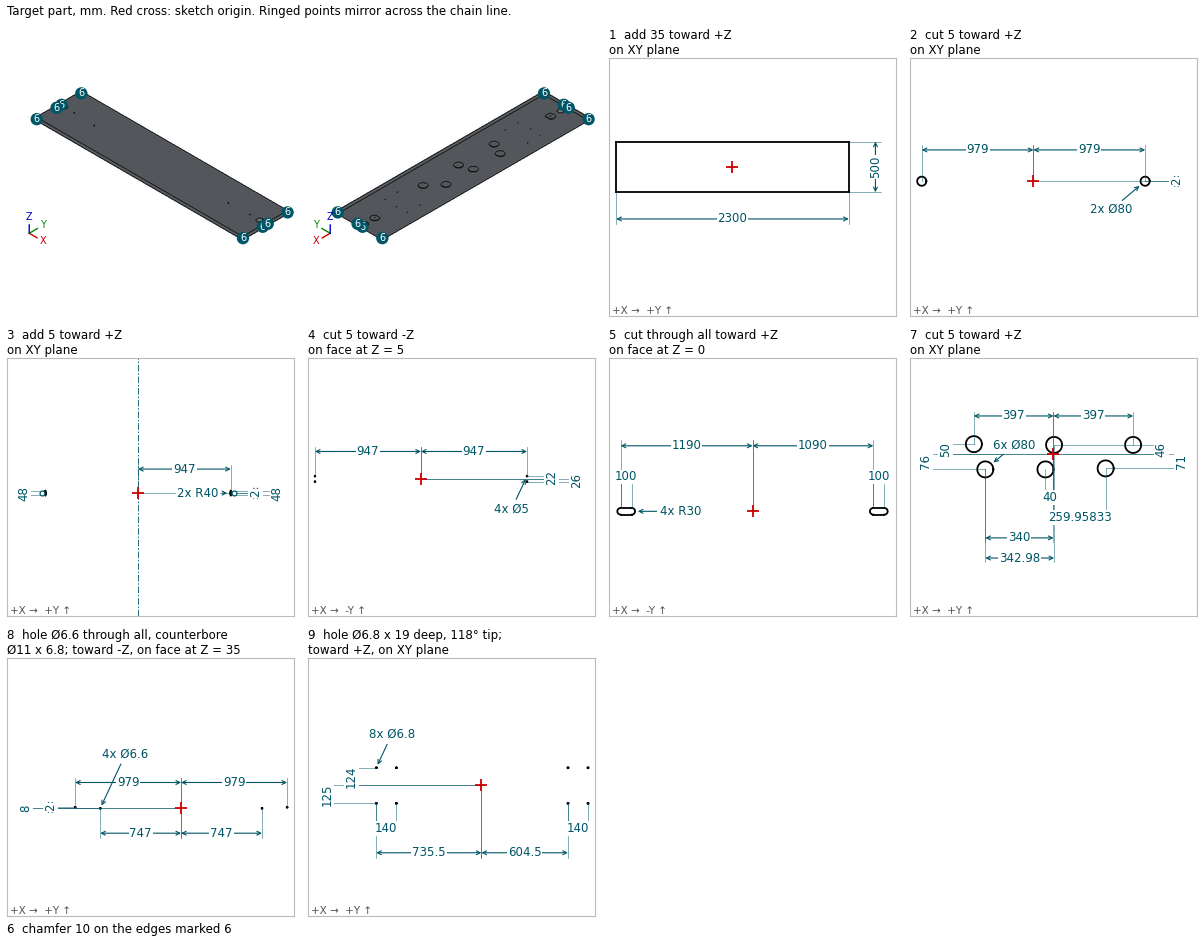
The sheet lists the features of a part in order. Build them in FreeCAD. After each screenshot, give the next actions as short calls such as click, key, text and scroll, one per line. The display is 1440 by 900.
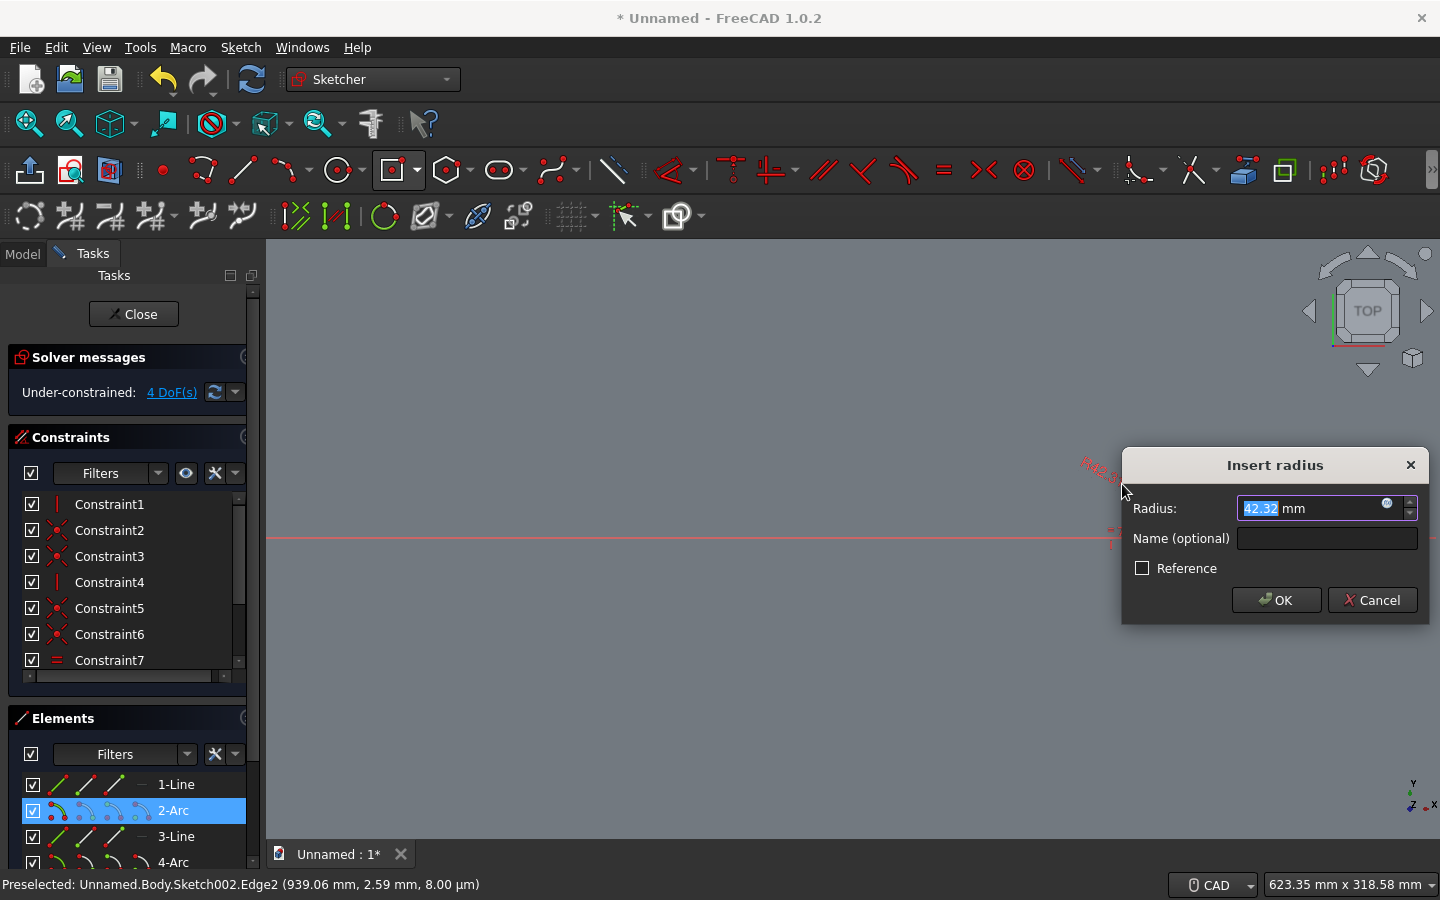
text(40)
key(Return)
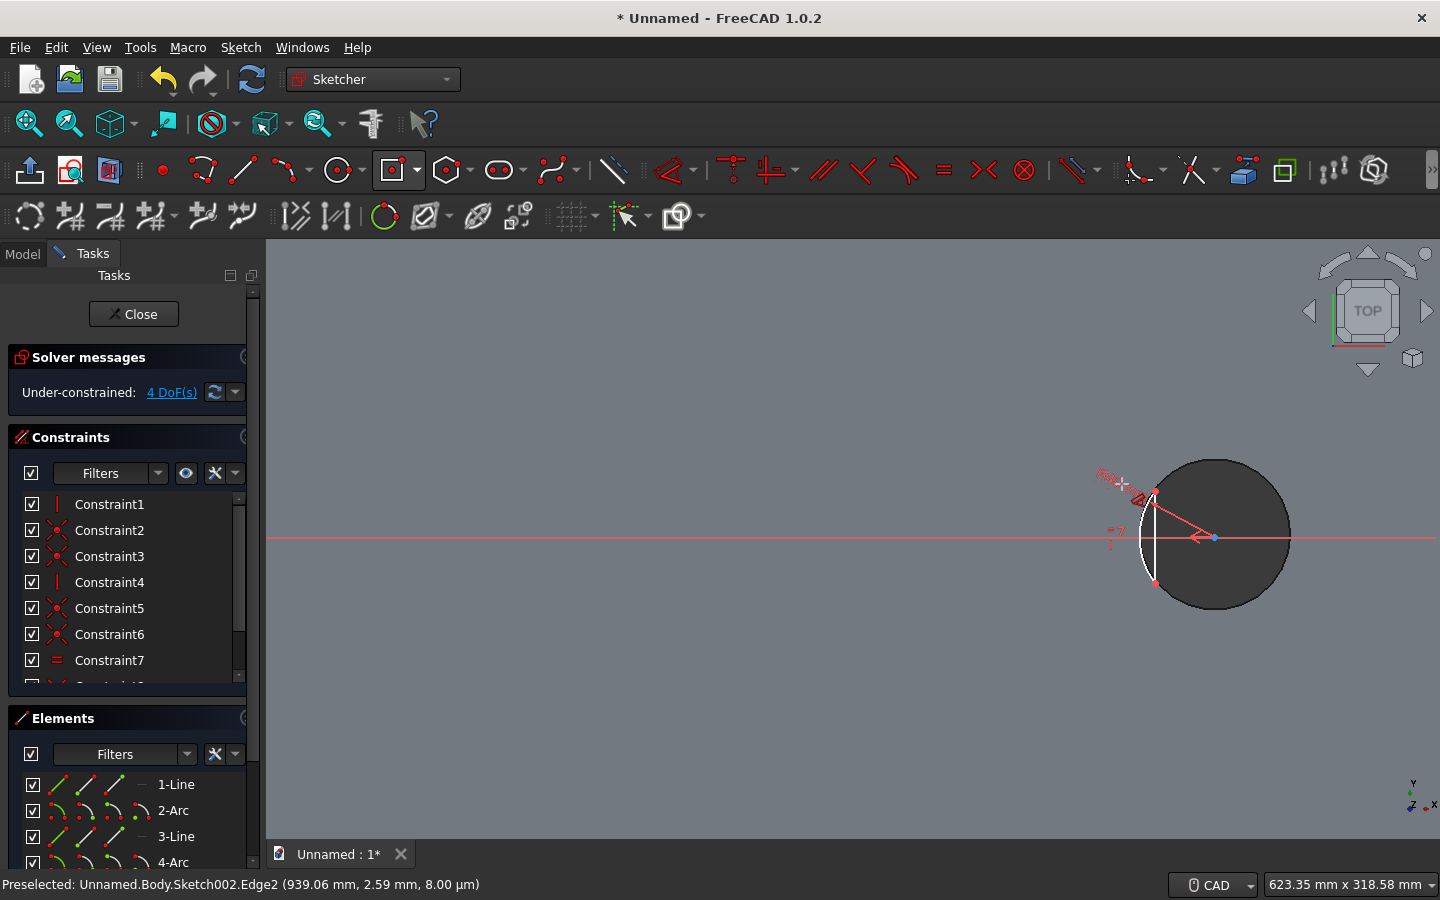
click(1155, 519)
click(1189, 516)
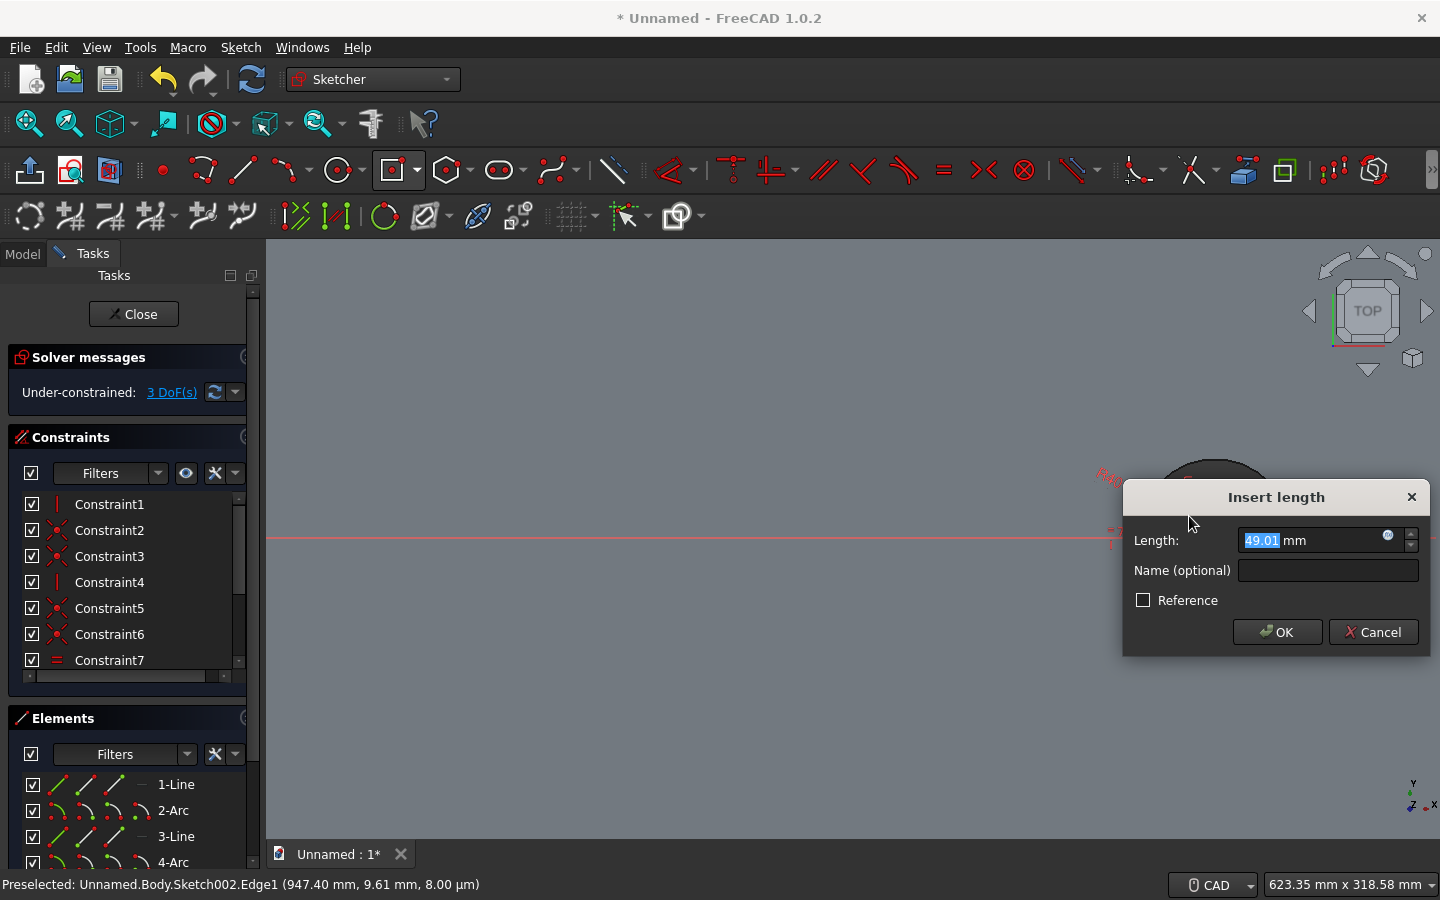
text(48)
key(Return)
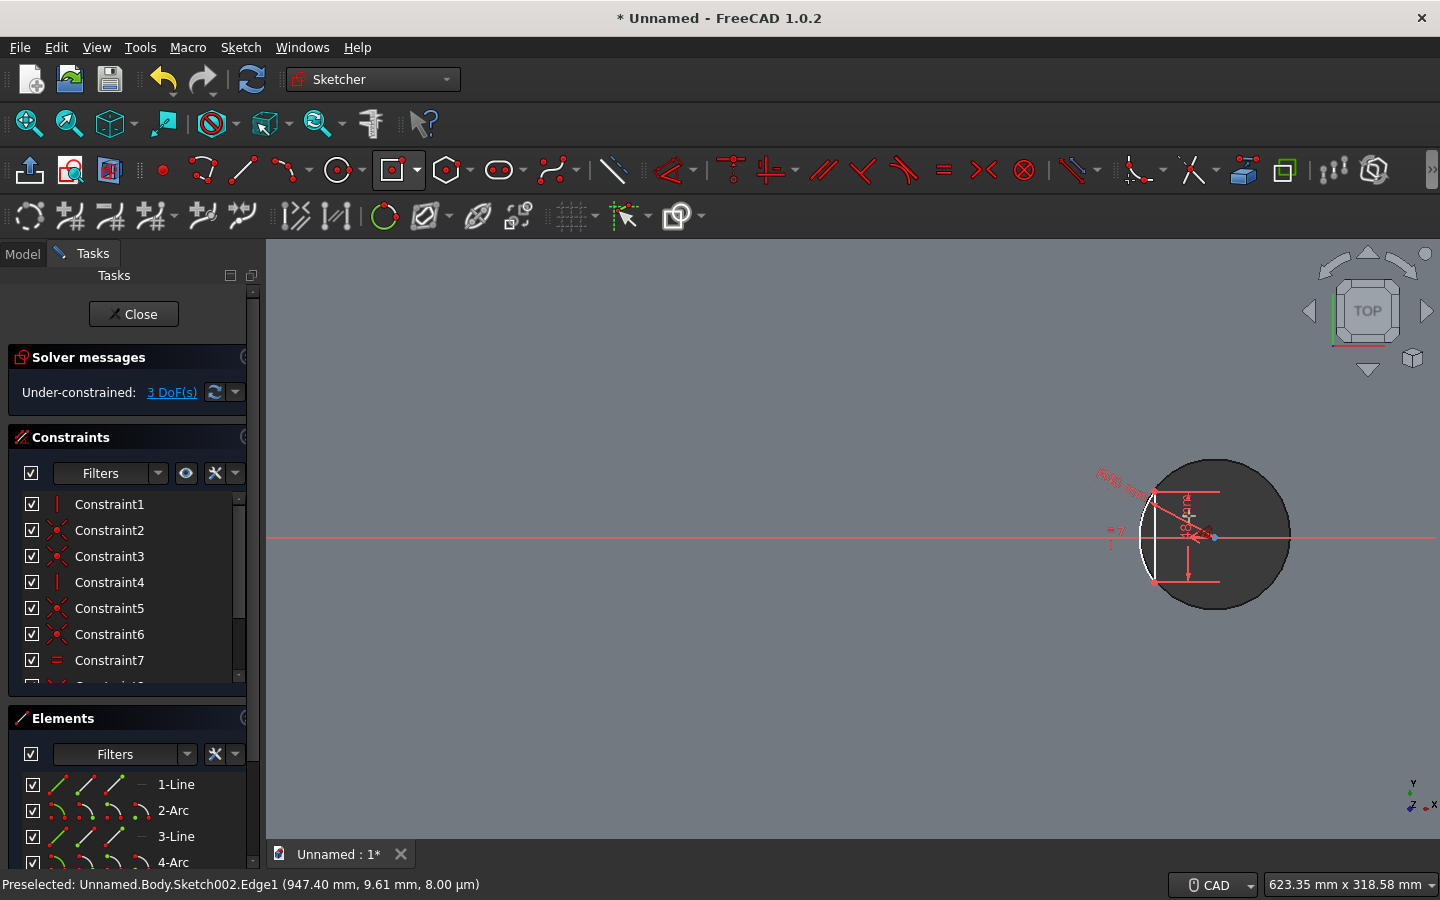
scroll(1142, 540, down, 8)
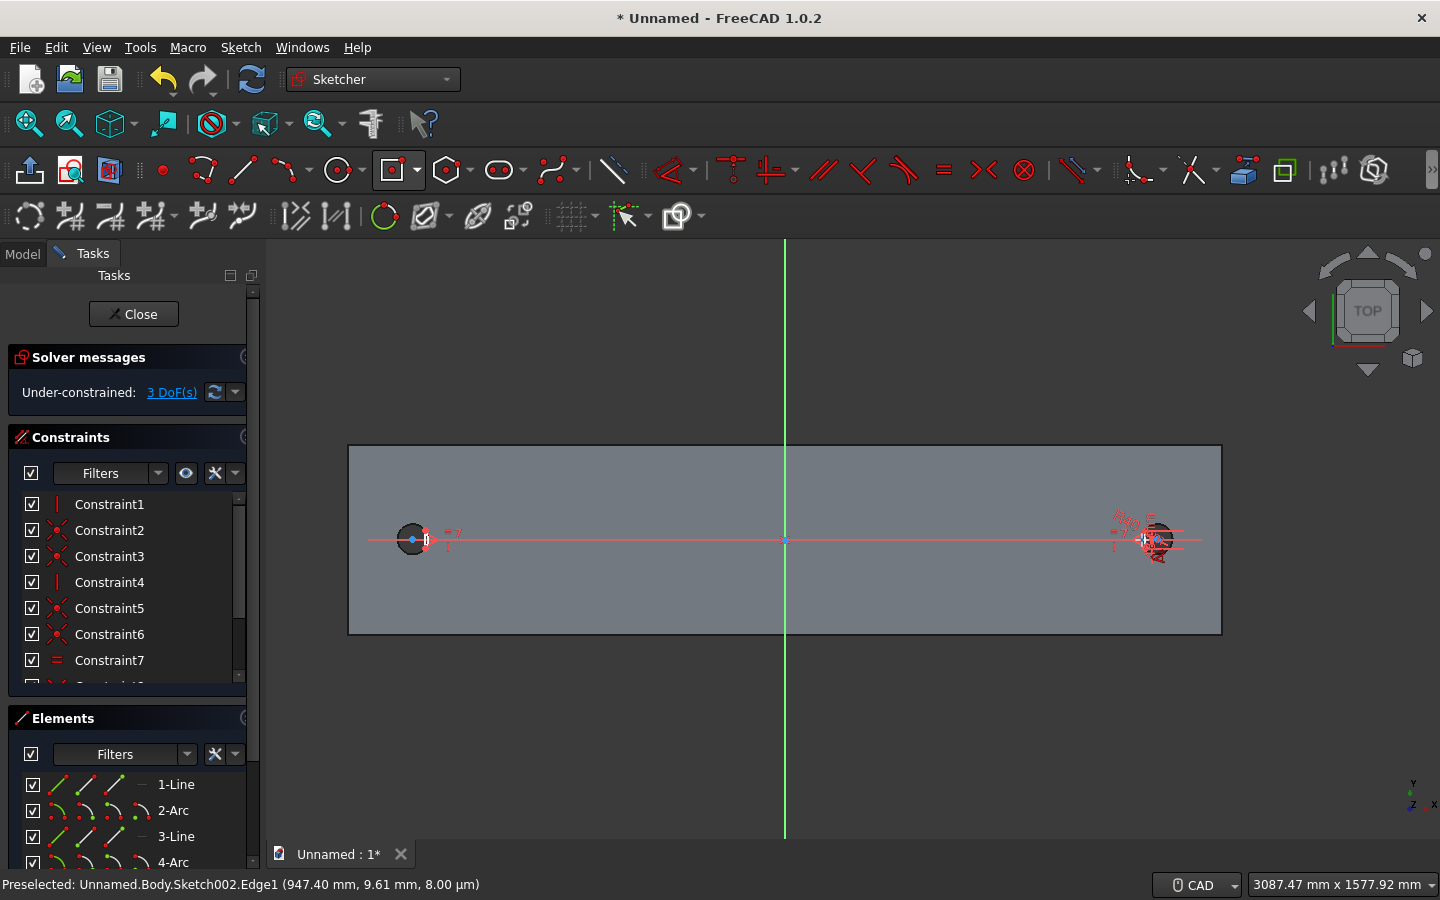
scroll(425, 543, up, 9)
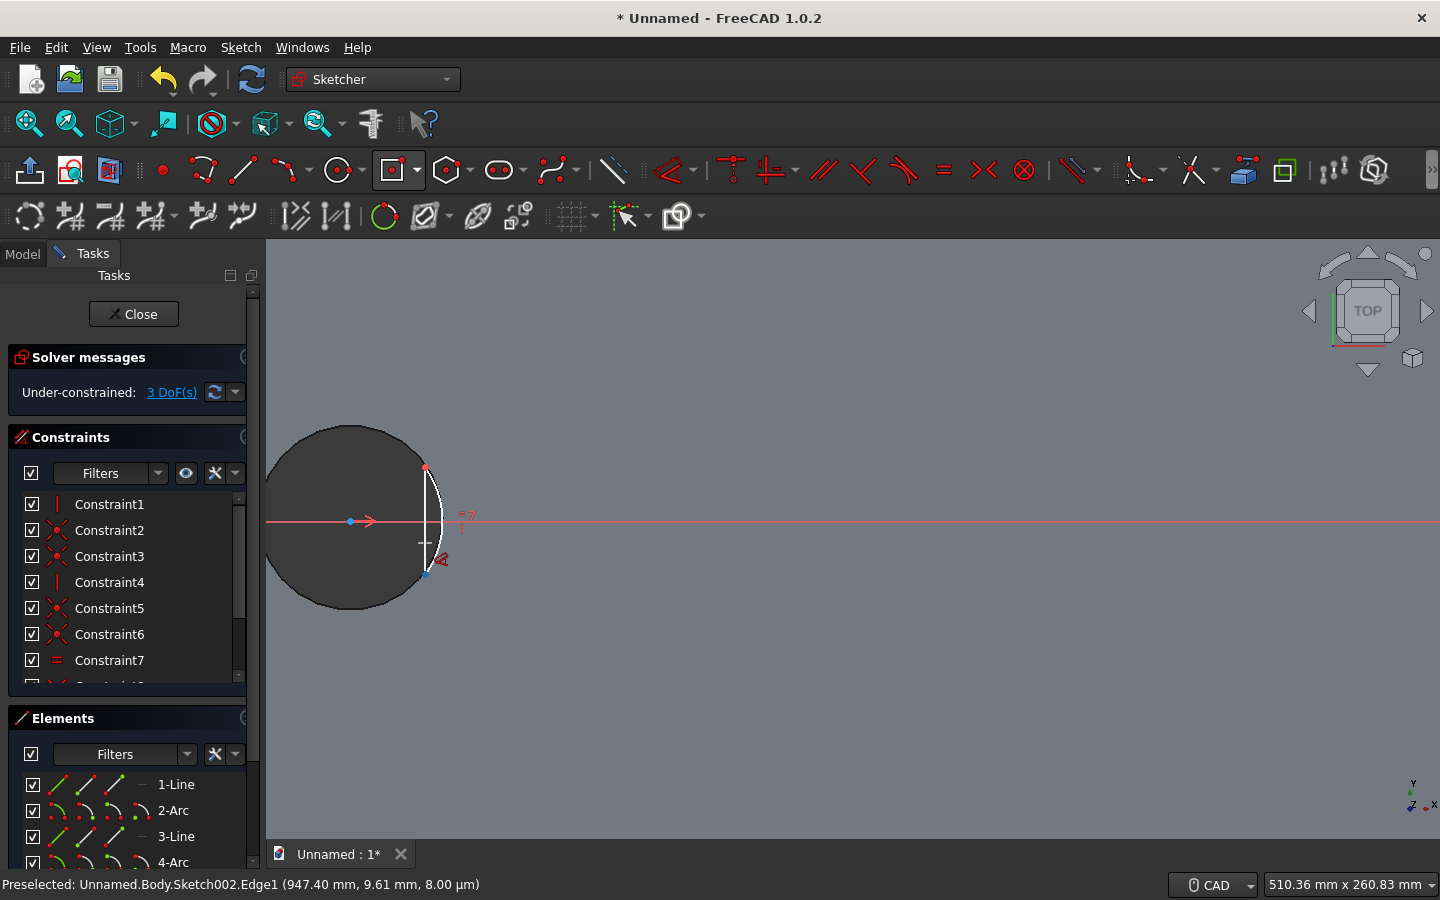
click(425, 543)
click(391, 497)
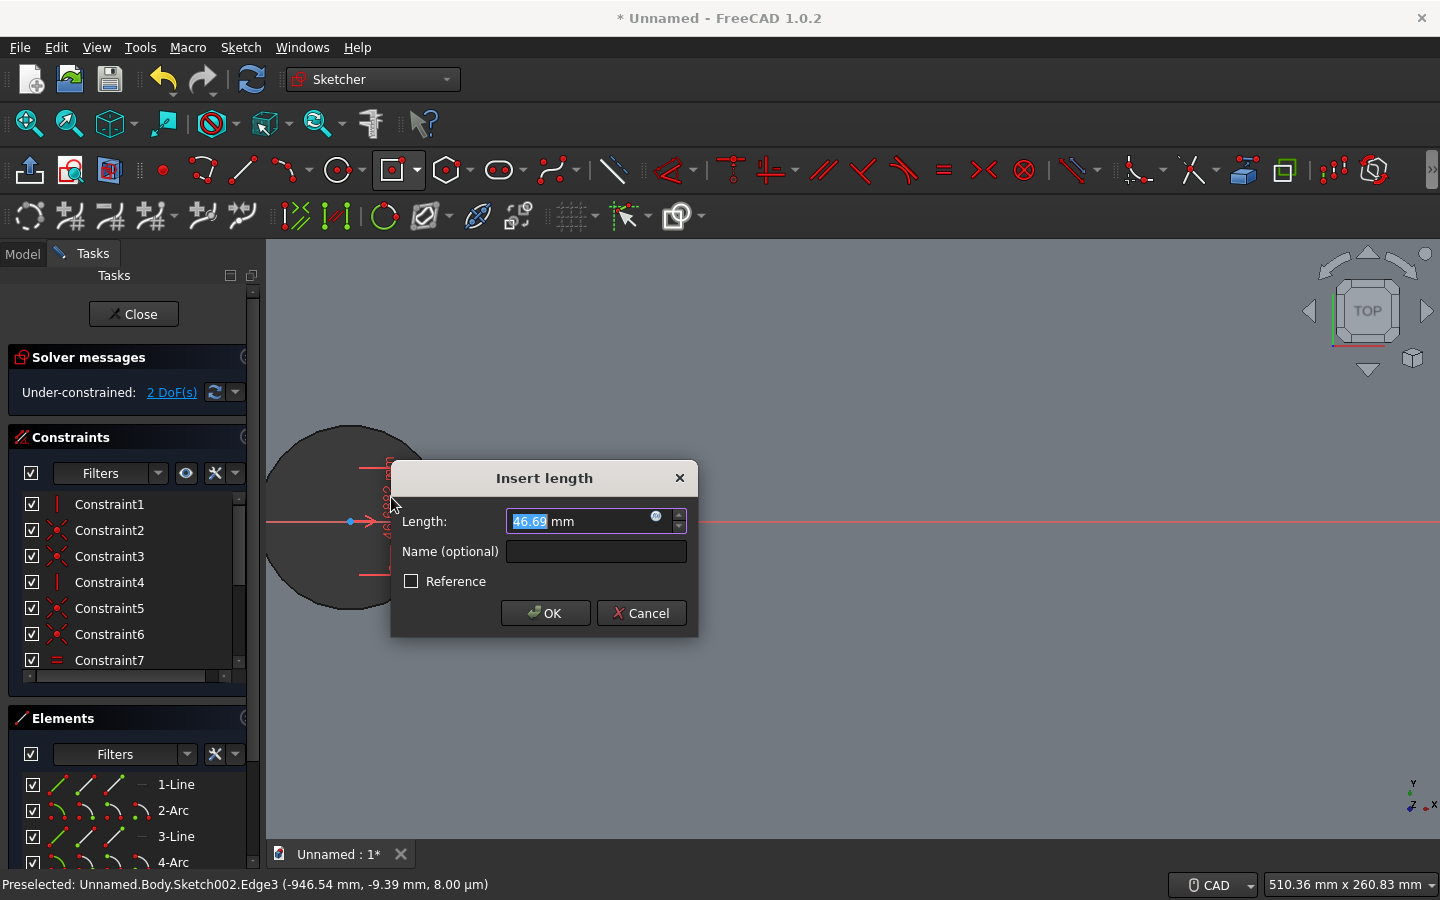
text(48)
key(Return)